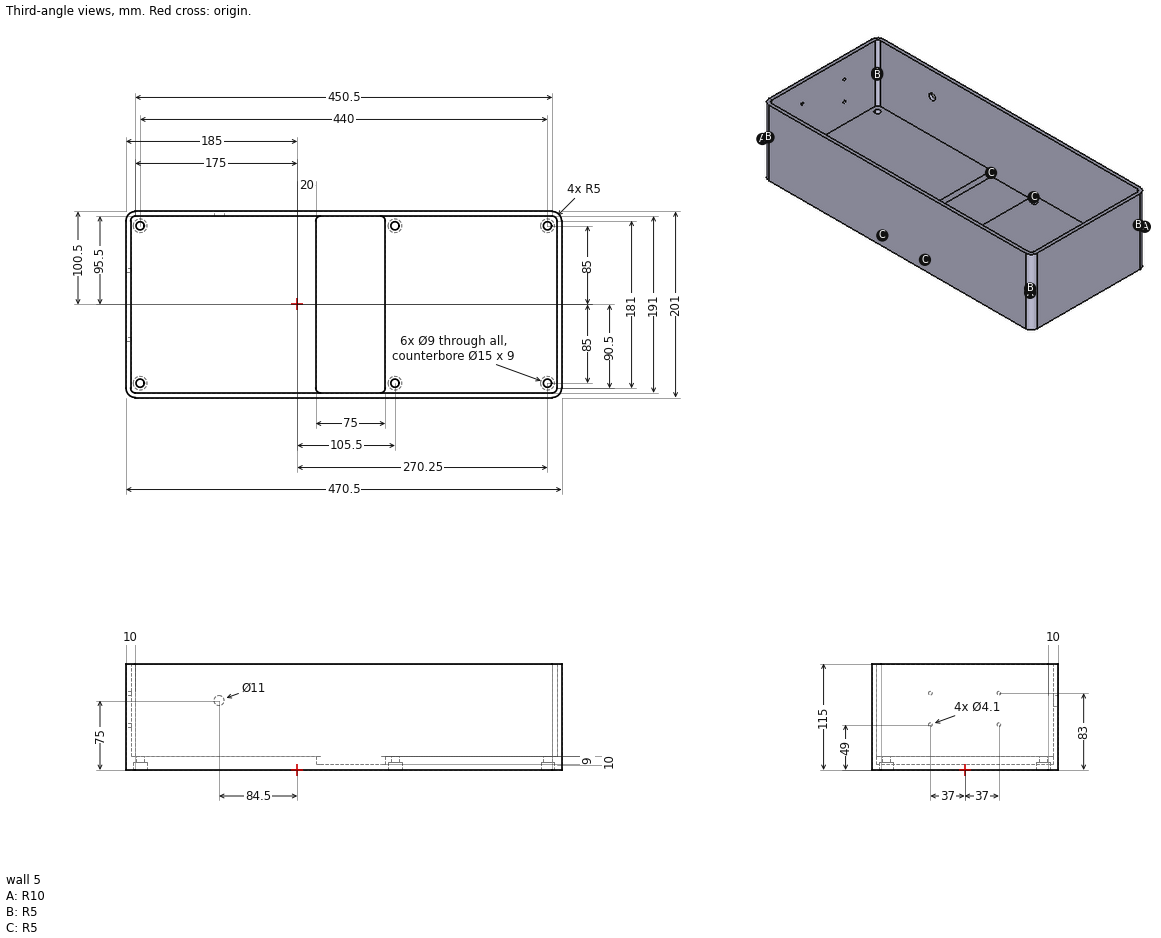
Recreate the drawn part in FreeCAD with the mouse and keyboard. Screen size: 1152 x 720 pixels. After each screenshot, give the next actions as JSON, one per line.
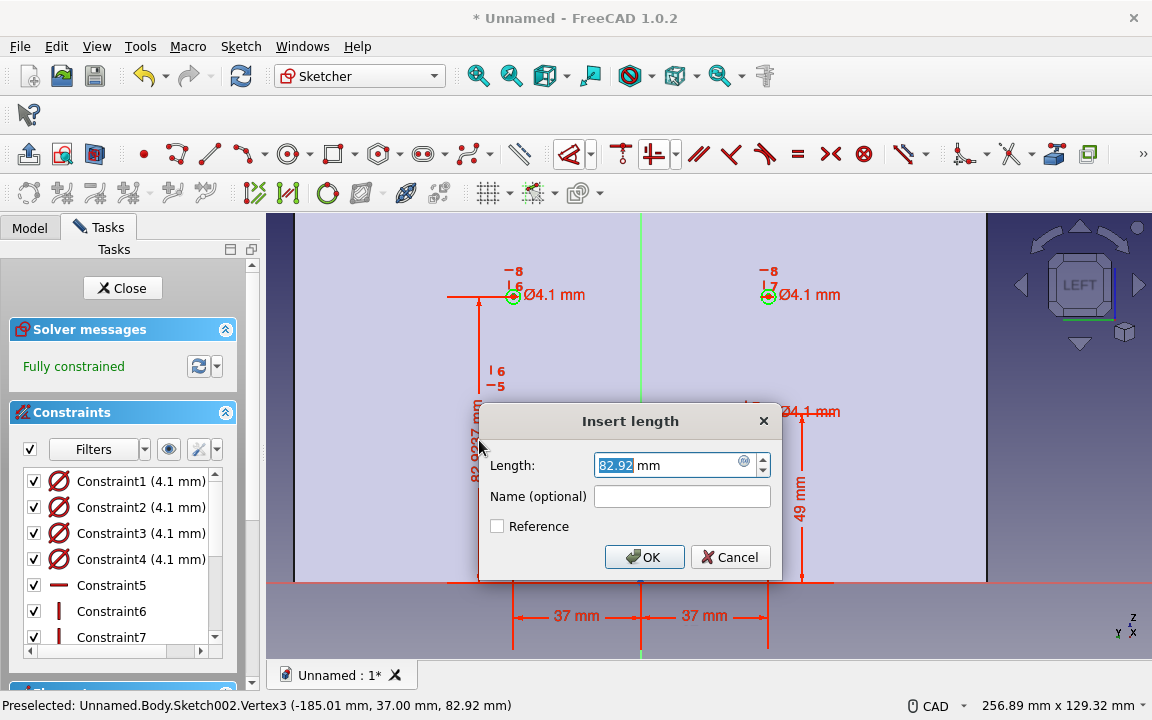
{"action": "type", "text": "83"}
{"action": "key", "text": "Return"}
{"action": "key", "text": "Escape"}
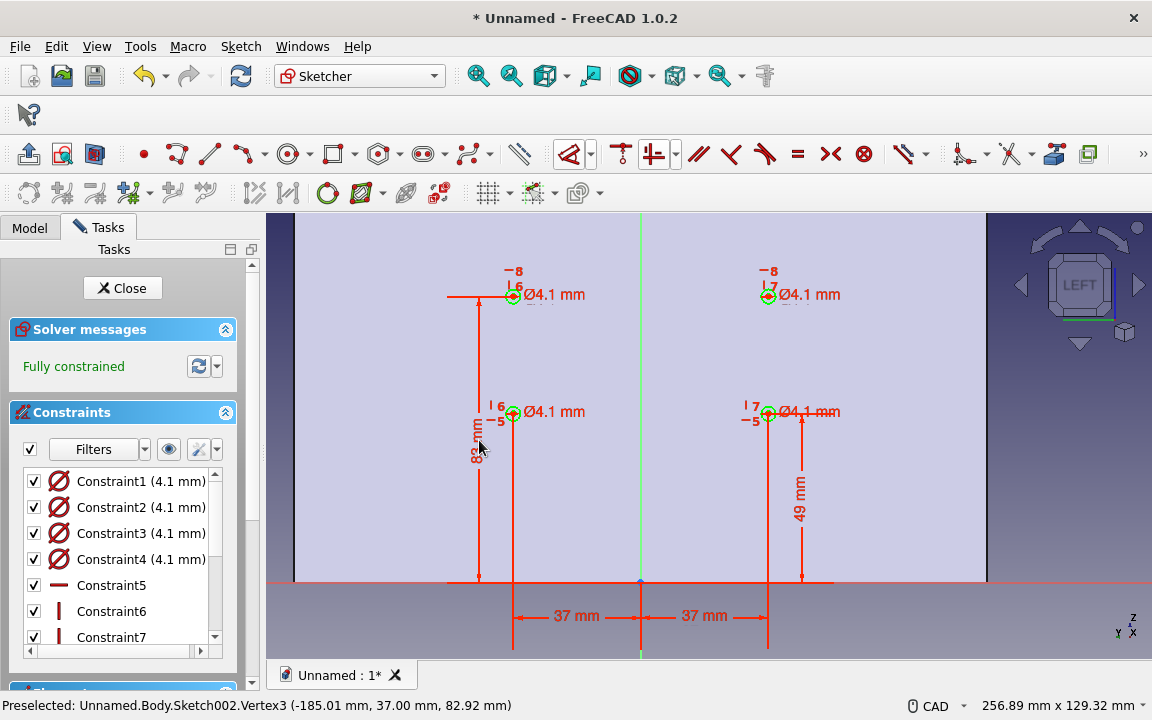
{"action": "left_click", "coordinate": [123, 288]}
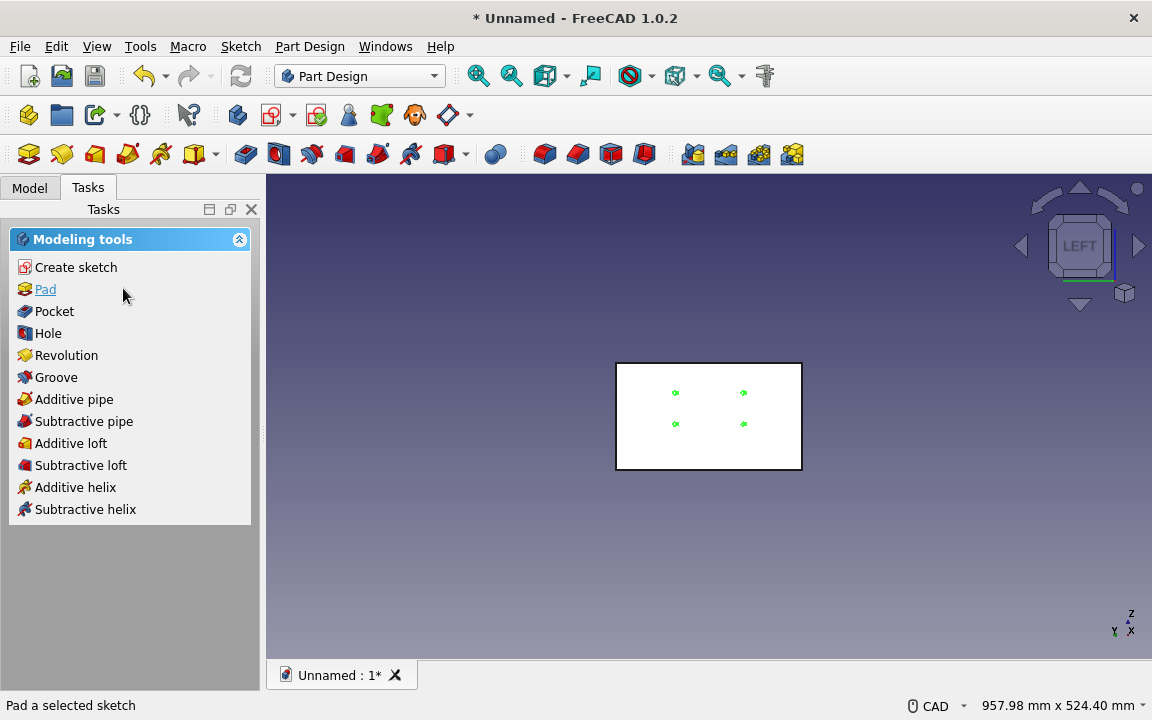
{"action": "left_click", "coordinate": [246, 154]}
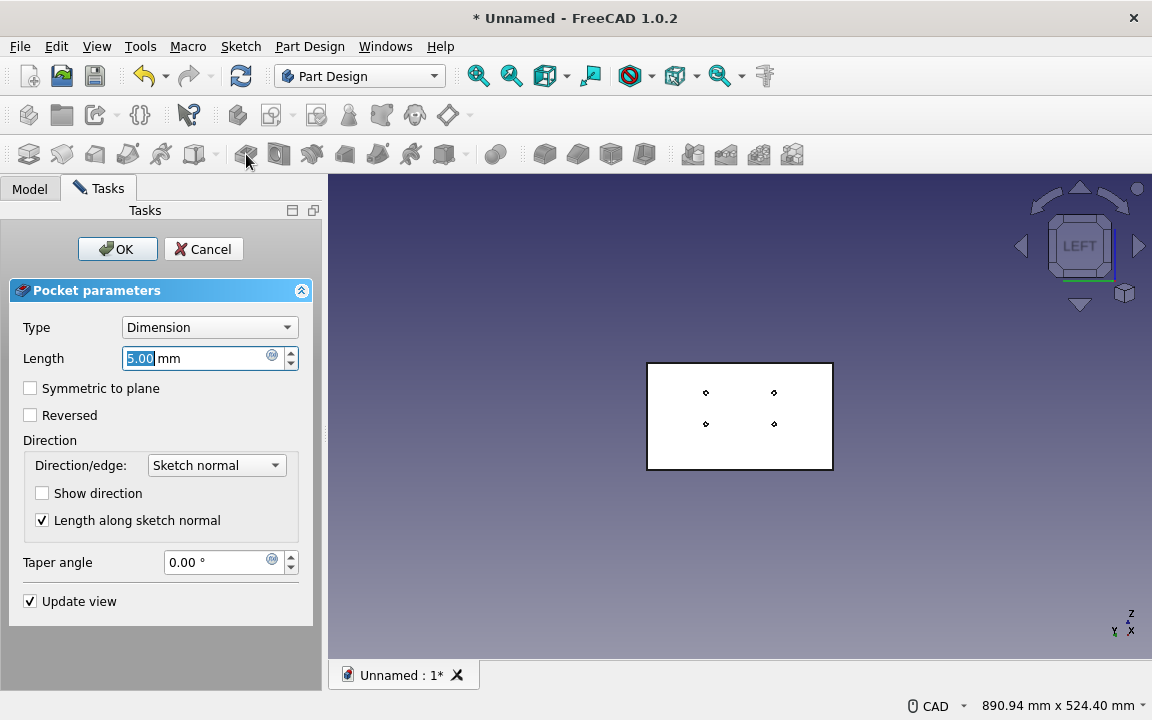
{"action": "type", "text": "10"}
{"action": "key", "text": "Tab"}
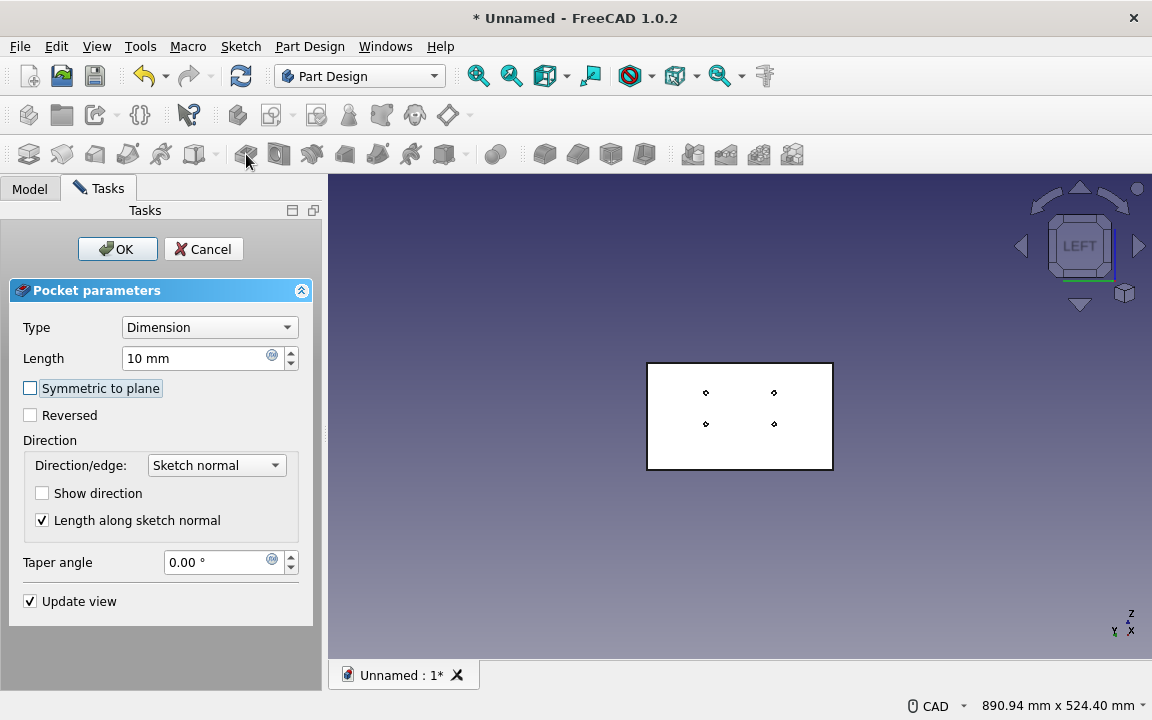
{"action": "left_click", "coordinate": [118, 249]}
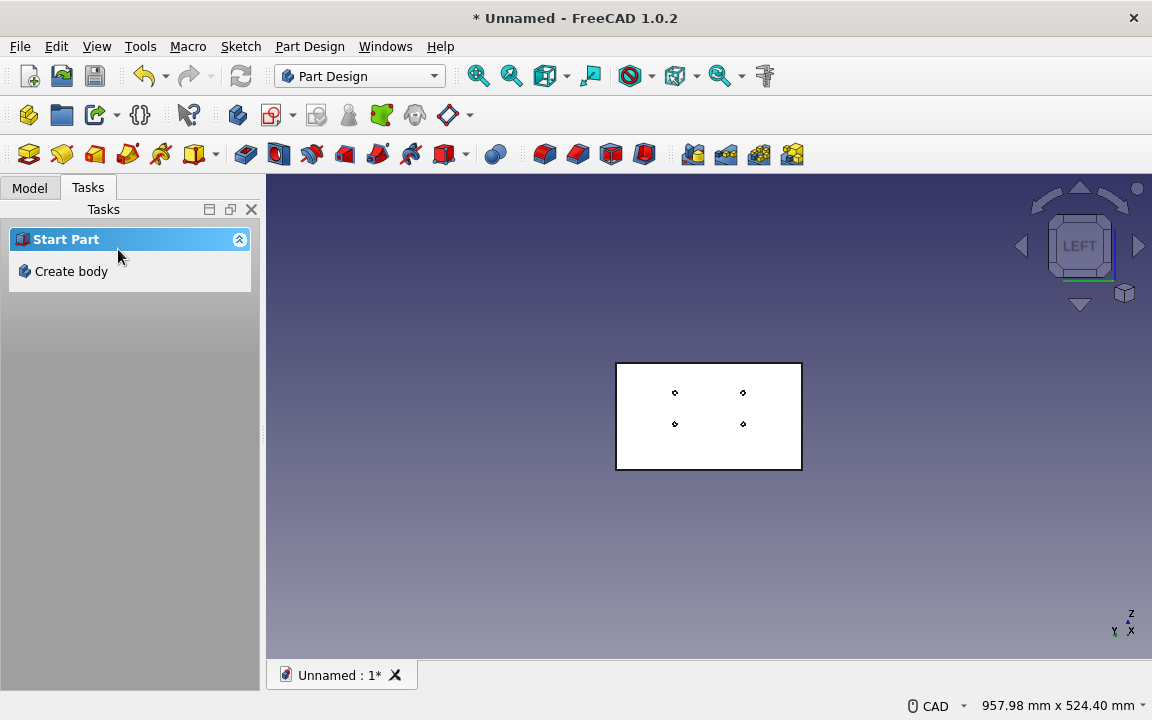
{"action": "key", "text": "v f"}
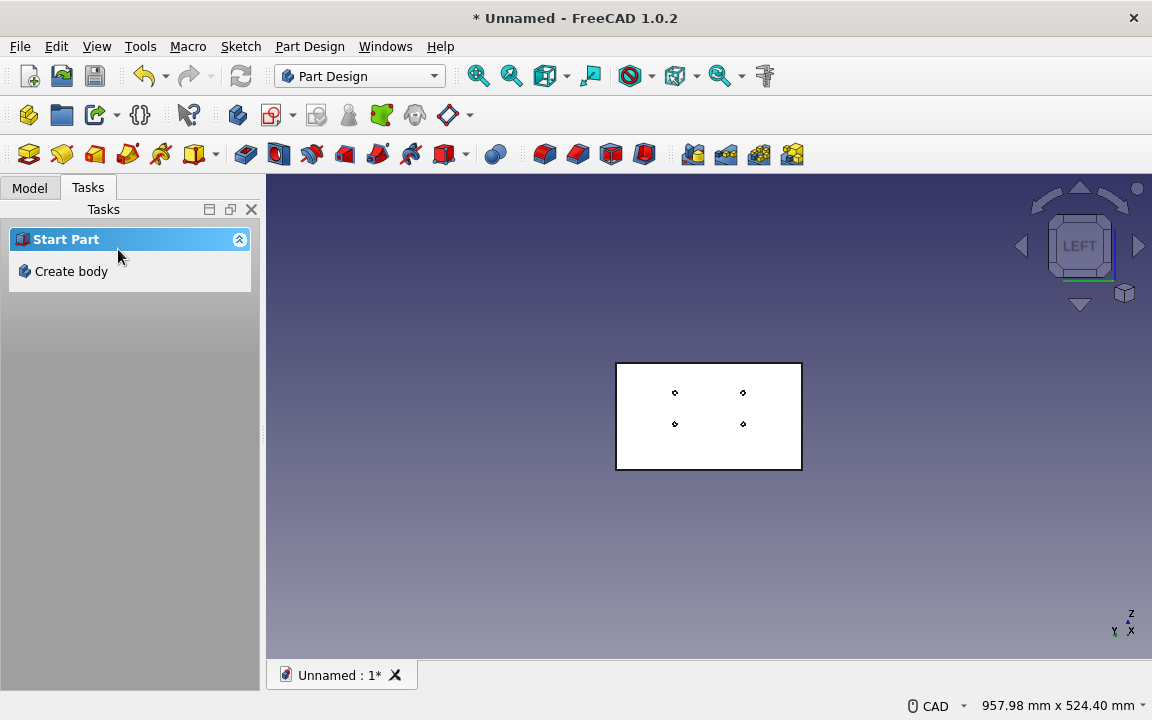
{"action": "left_click", "coordinate": [802, 415]}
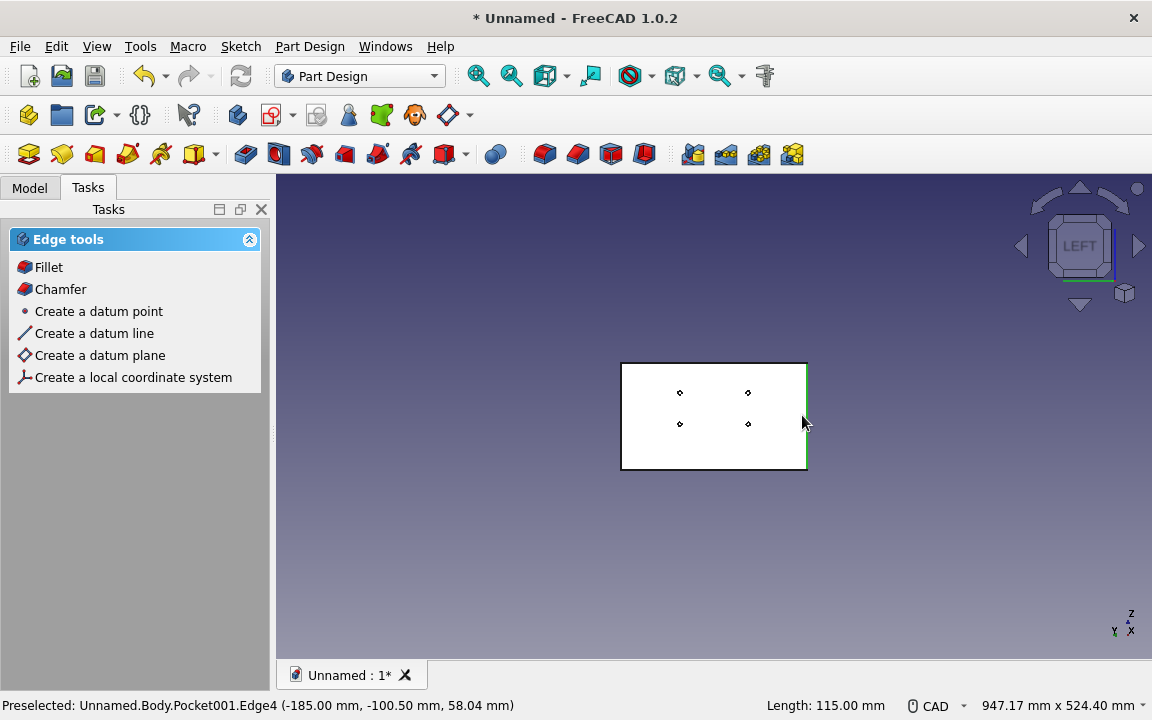
{"action": "left_click", "coordinate": [621, 415], "text": "ctrl"}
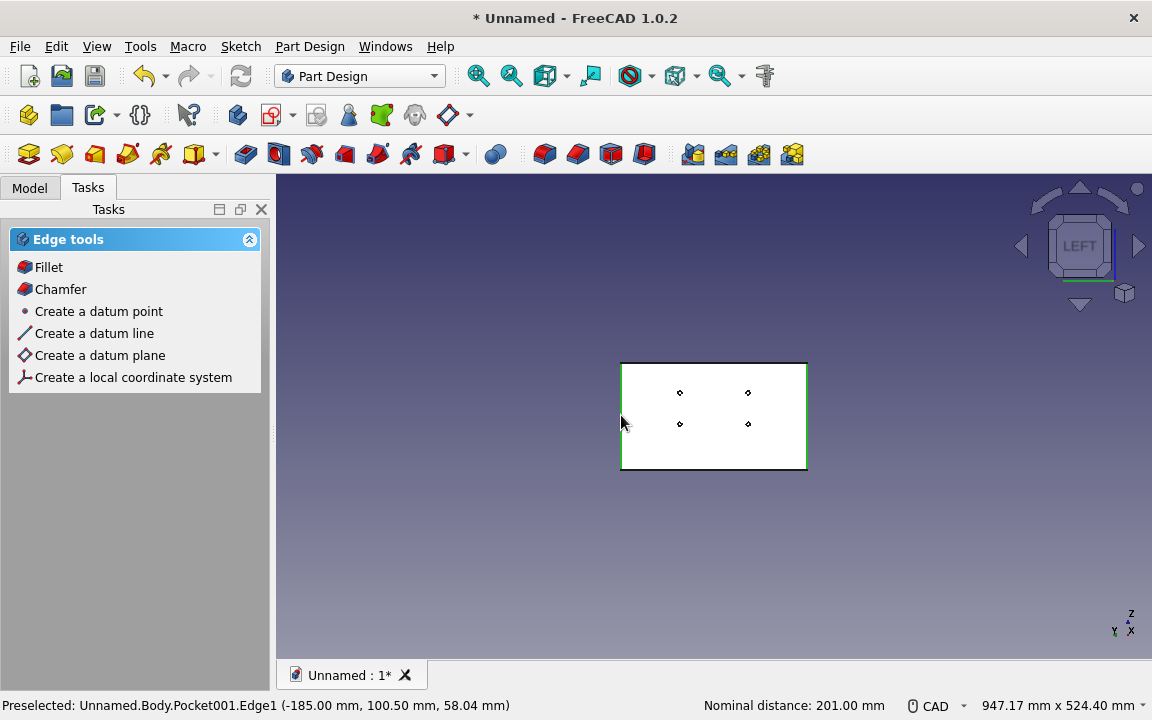
{"action": "key", "text": "0"}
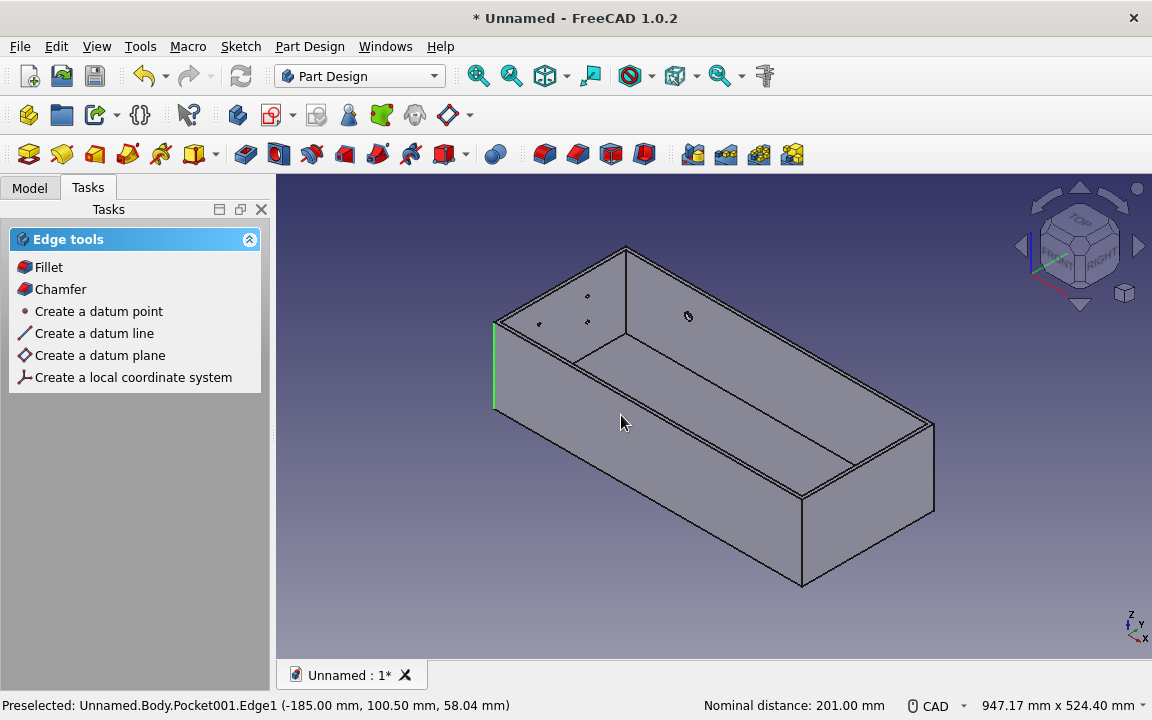
{"action": "left_click", "coordinate": [802, 542], "text": "ctrl"}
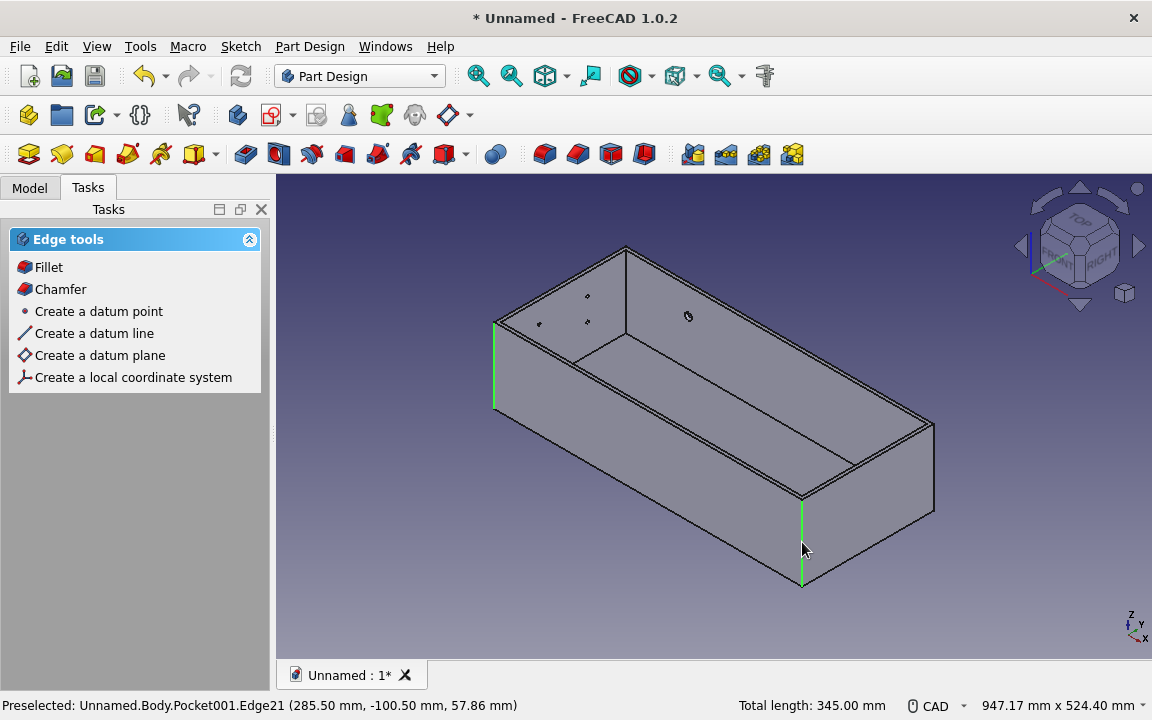
{"action": "key", "text": "2"}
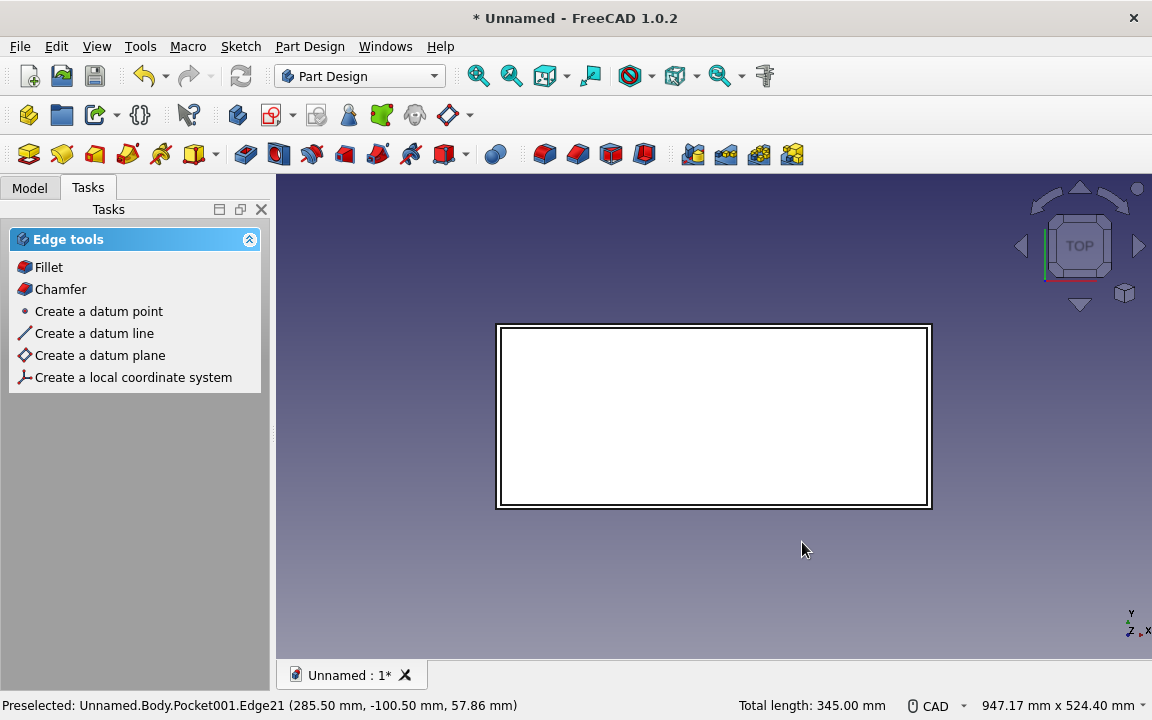
{"action": "key", "text": "1"}